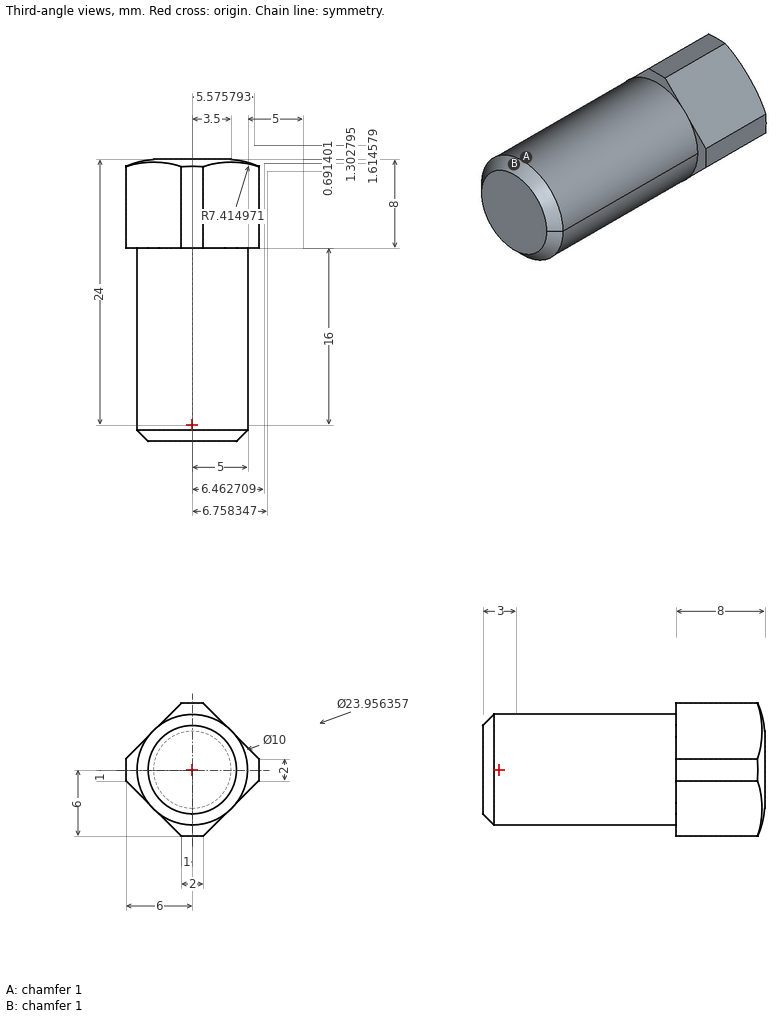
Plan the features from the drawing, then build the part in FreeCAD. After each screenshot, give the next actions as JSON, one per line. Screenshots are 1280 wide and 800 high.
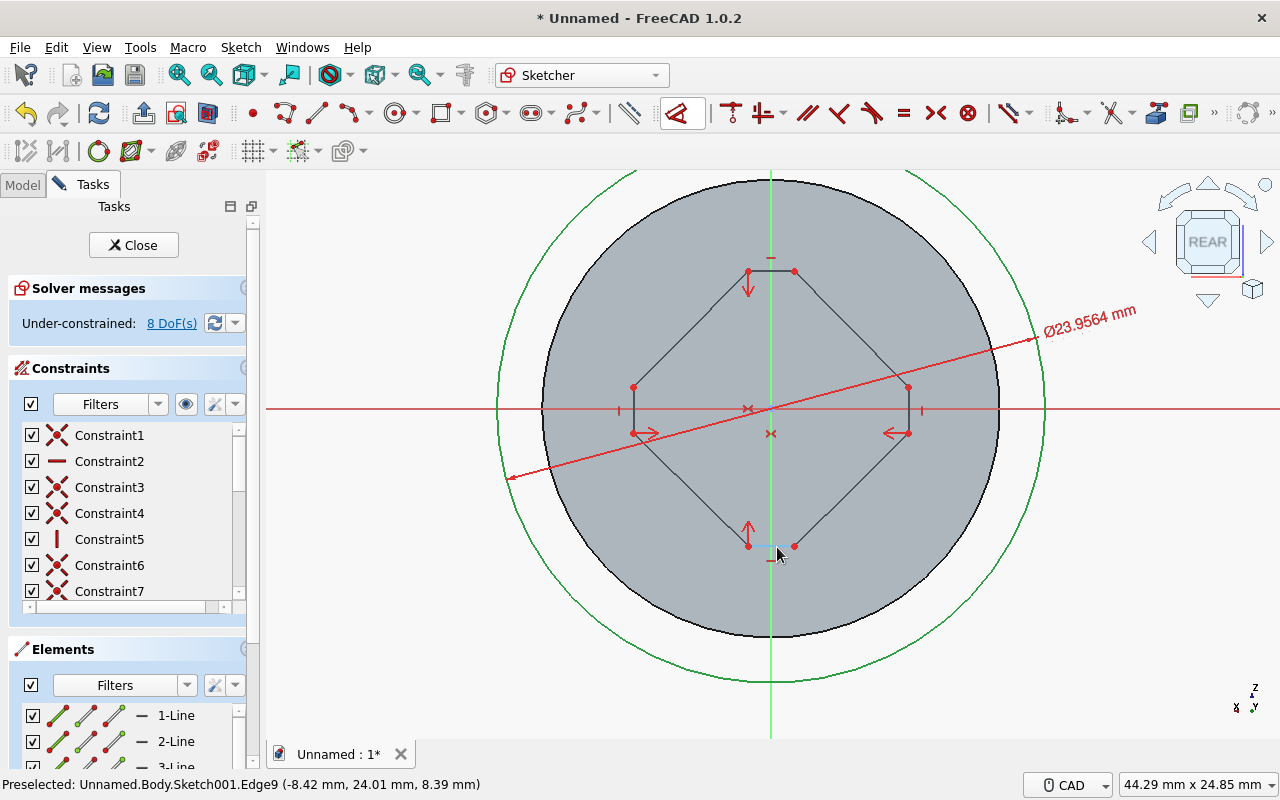
{"action": "left_click", "coordinate": [776, 546]}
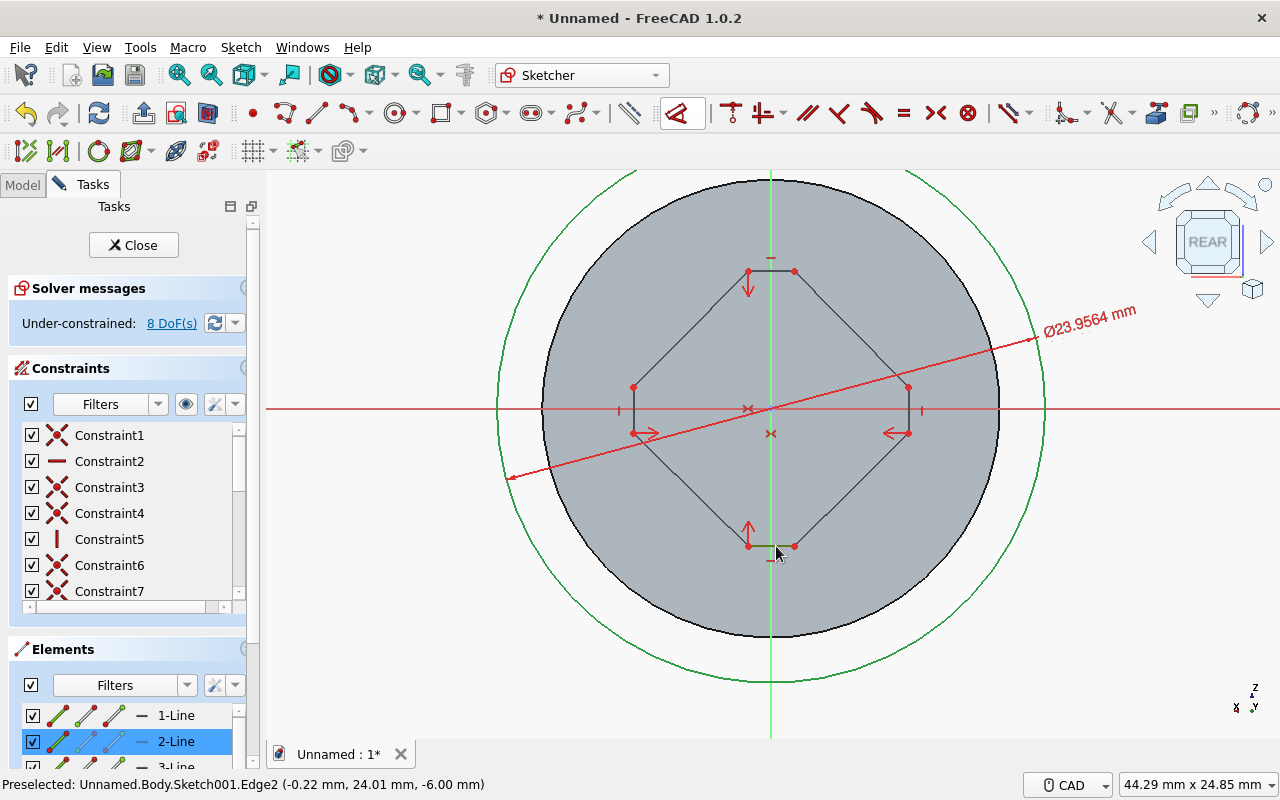
{"action": "key", "text": "l"}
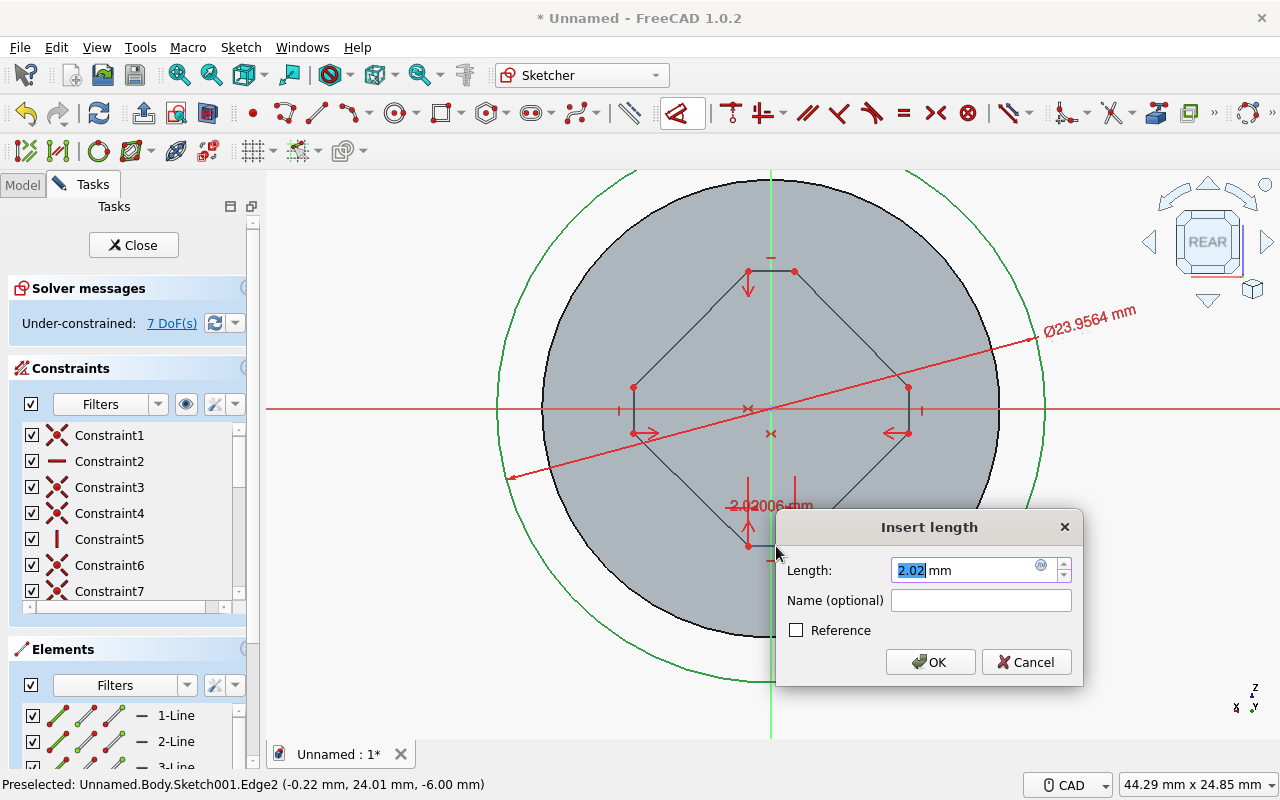
{"action": "type", "text": "2"}
{"action": "key", "text": "Return"}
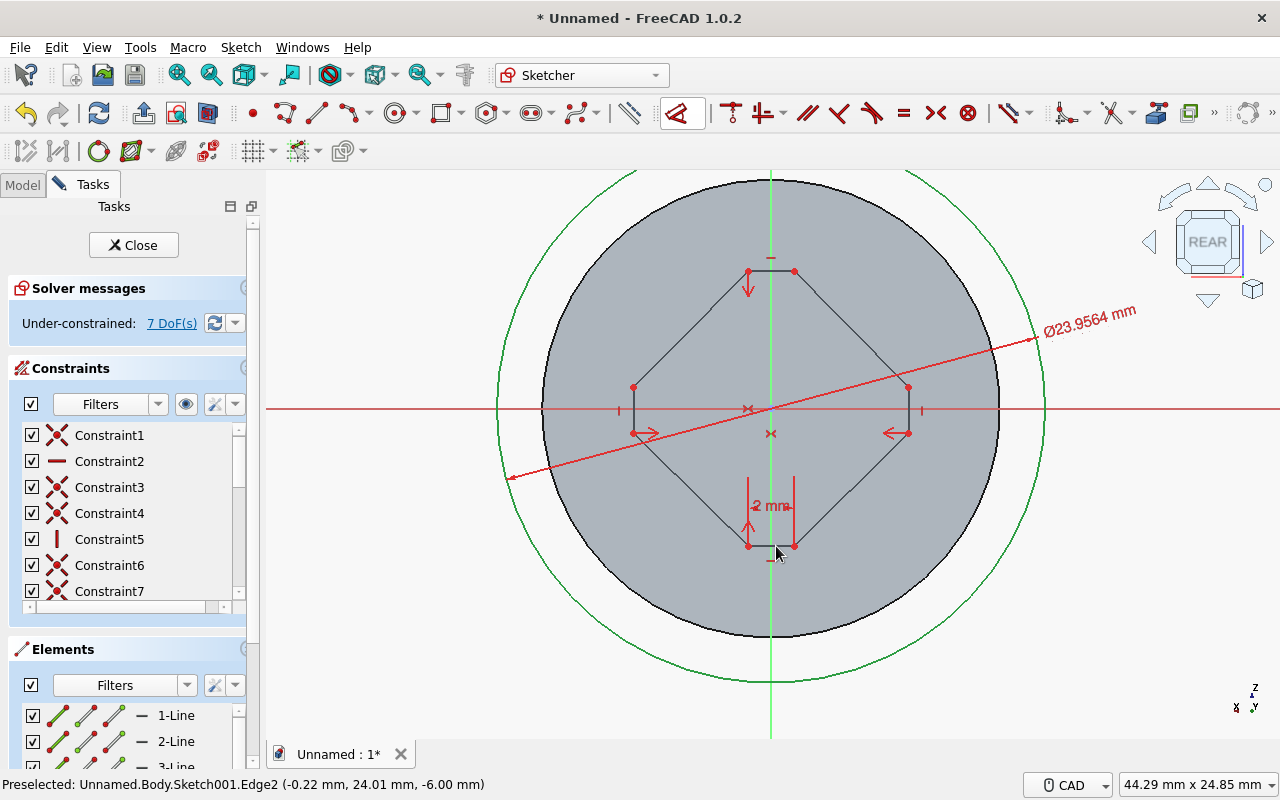
{"action": "scroll", "coordinate": [634, 419], "scroll_direction": "up", "scroll_amount": 2}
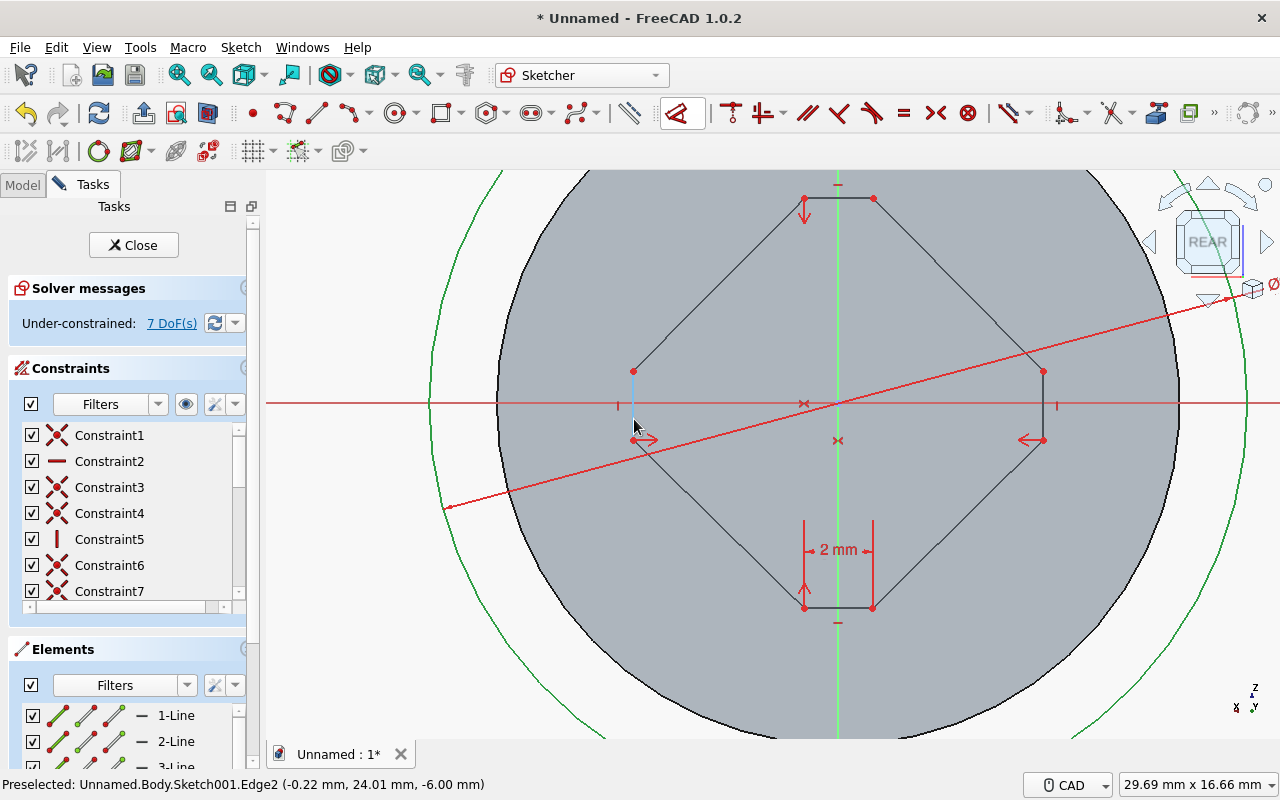
{"action": "left_click", "coordinate": [633, 419]}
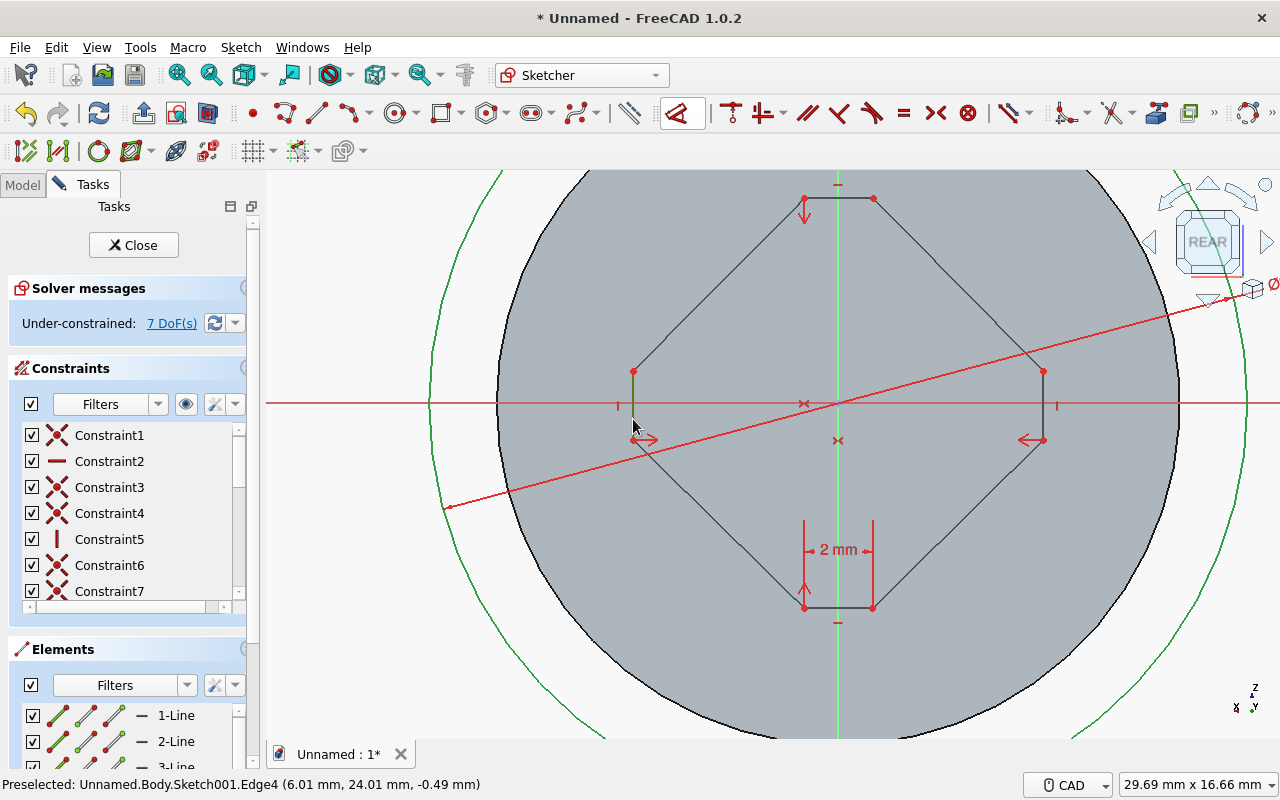
{"action": "left_click", "coordinate": [700, 114]}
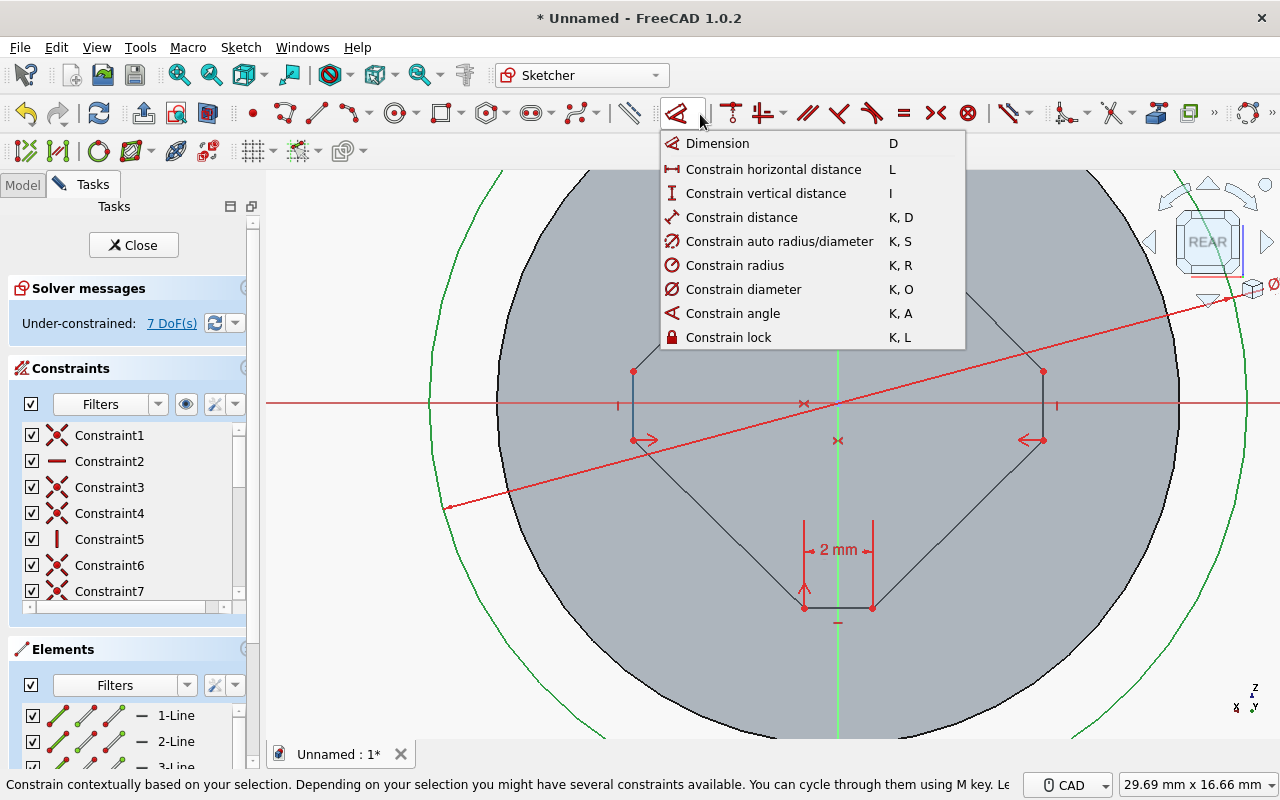
{"action": "left_click", "coordinate": [813, 193]}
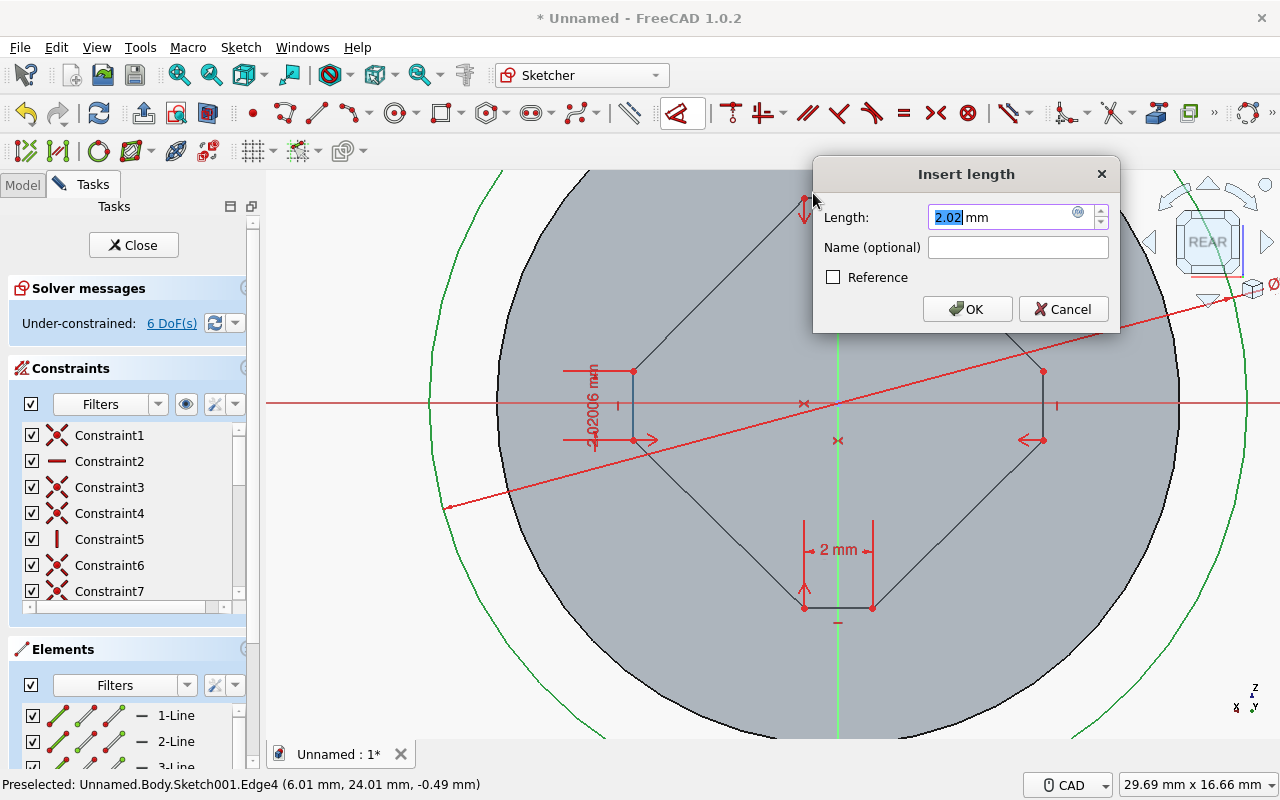
{"action": "type", "text": "2"}
{"action": "key", "text": "Return"}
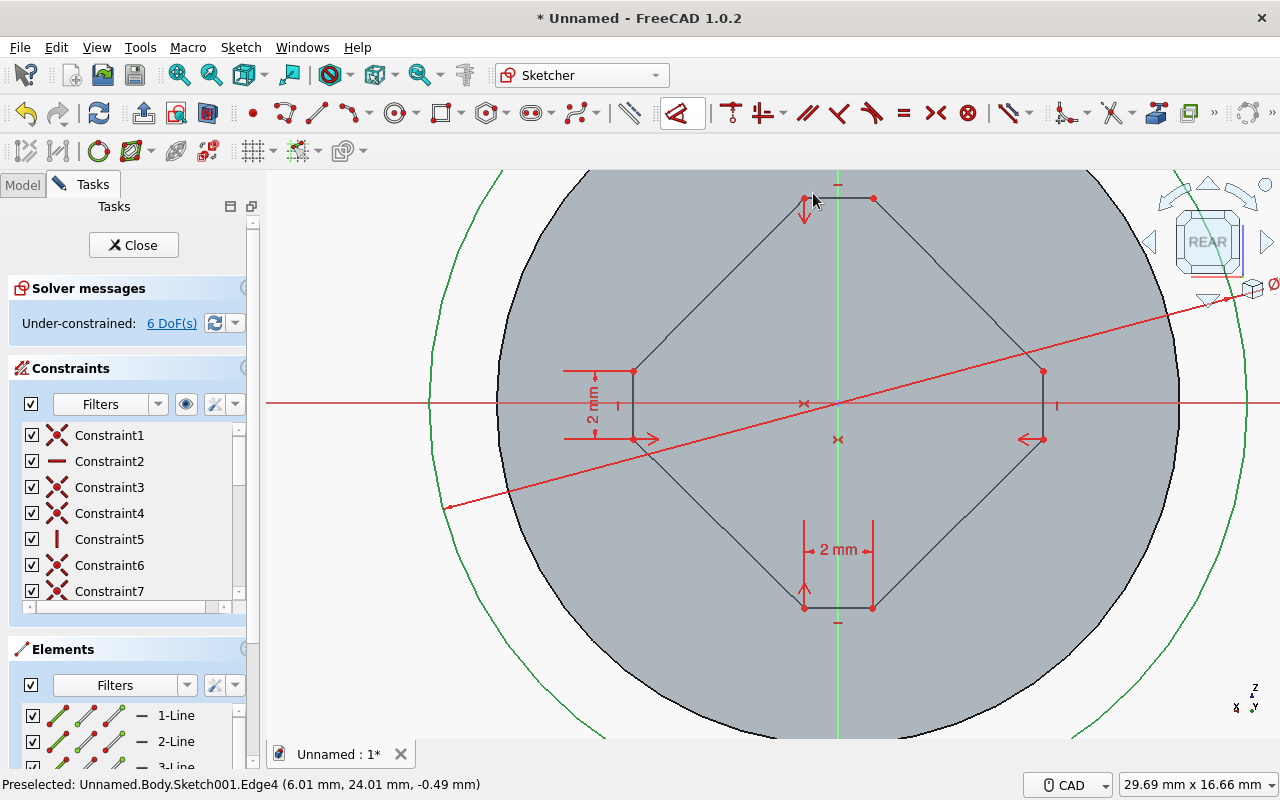
{"action": "left_click", "coordinate": [825, 198]}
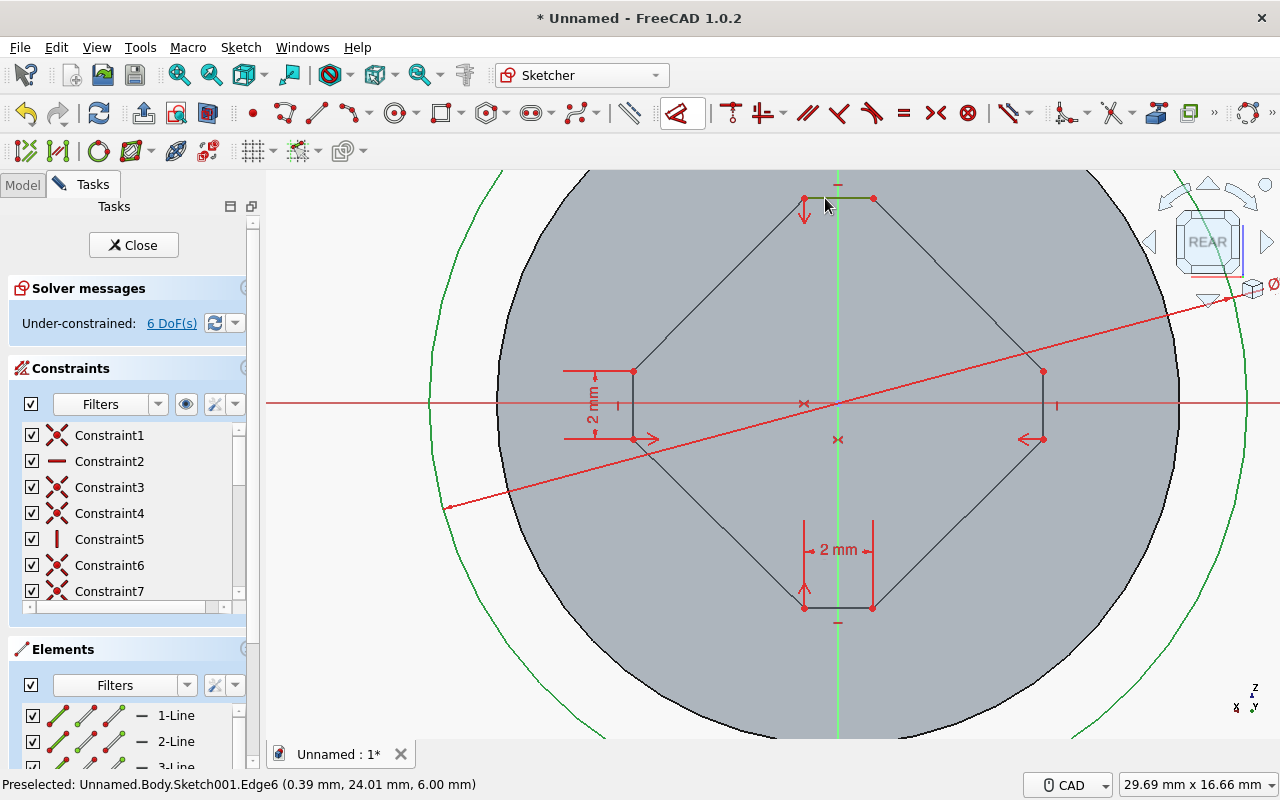
{"action": "key", "text": "l"}